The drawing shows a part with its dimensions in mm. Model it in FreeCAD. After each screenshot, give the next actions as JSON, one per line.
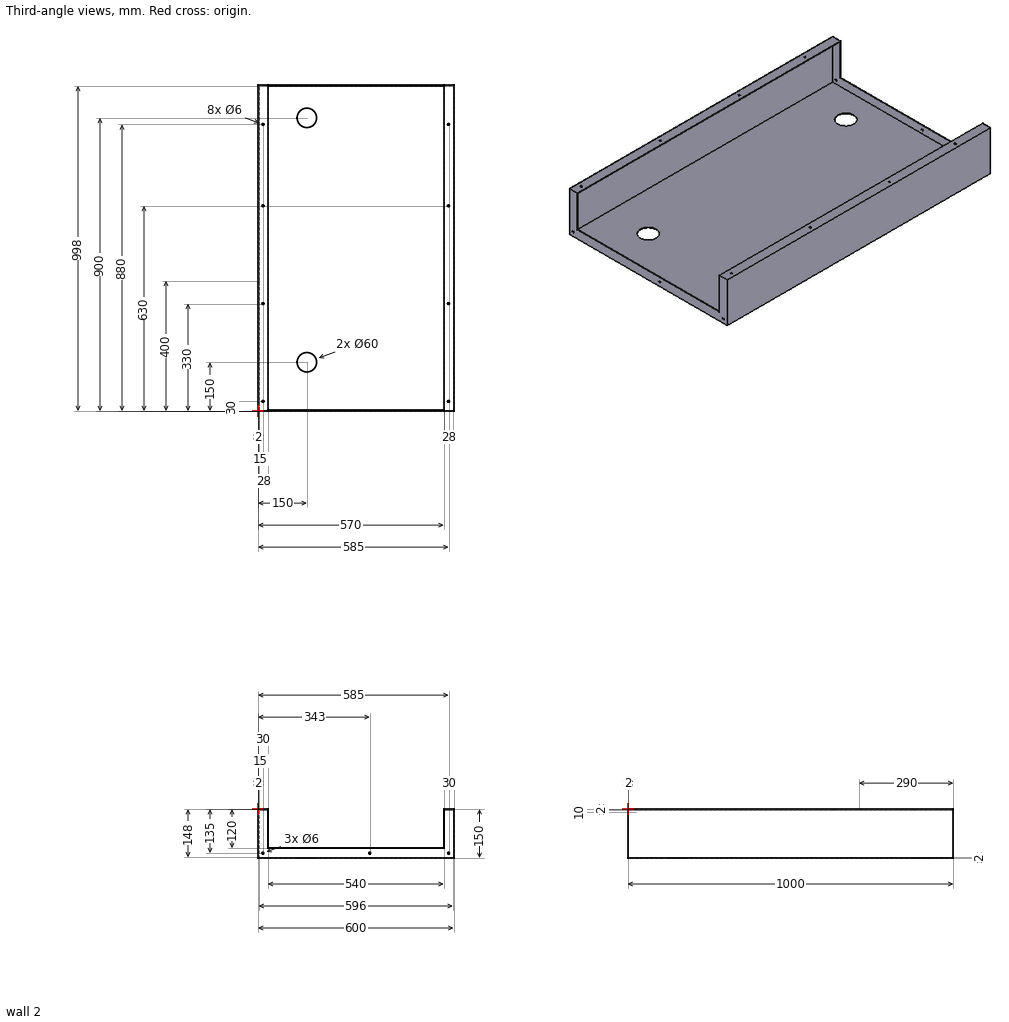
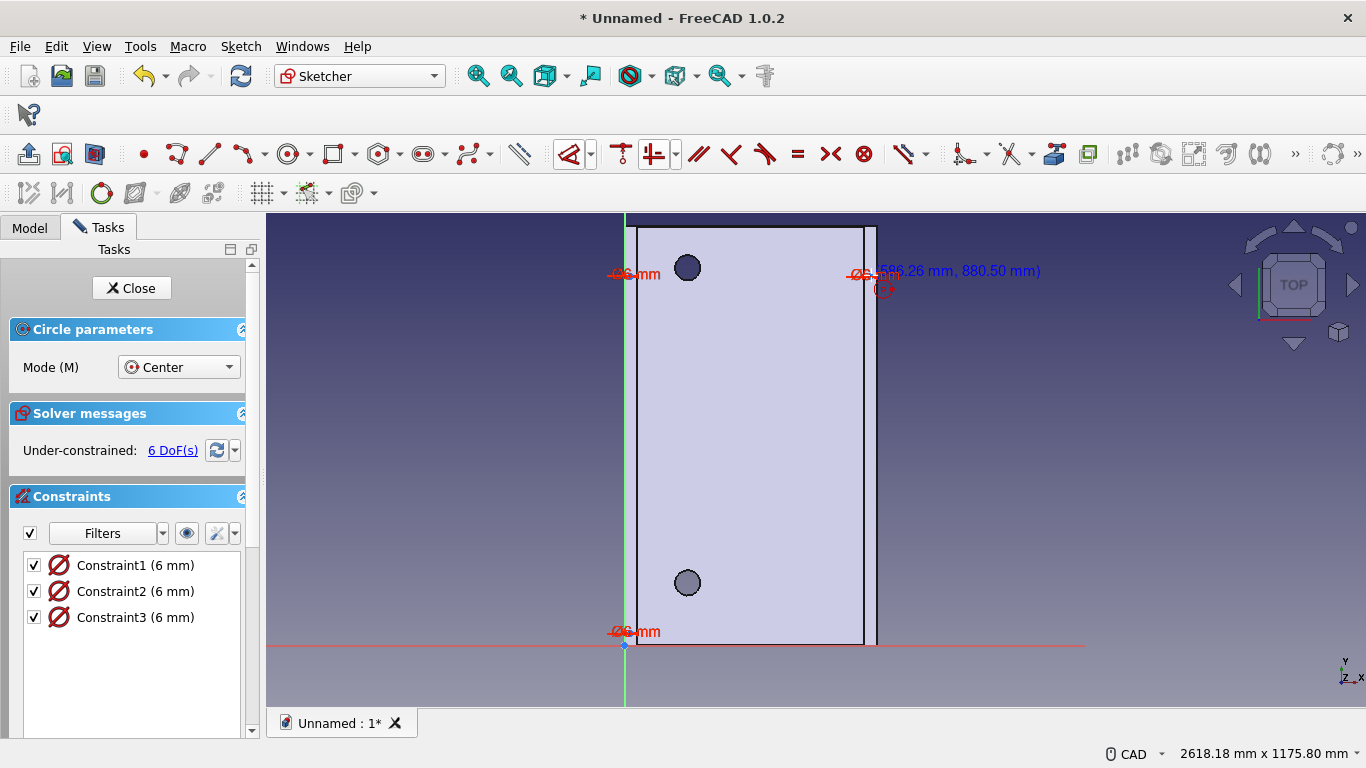
{"action": "scroll", "coordinate": [631, 507], "scroll_direction": "up", "scroll_amount": 15}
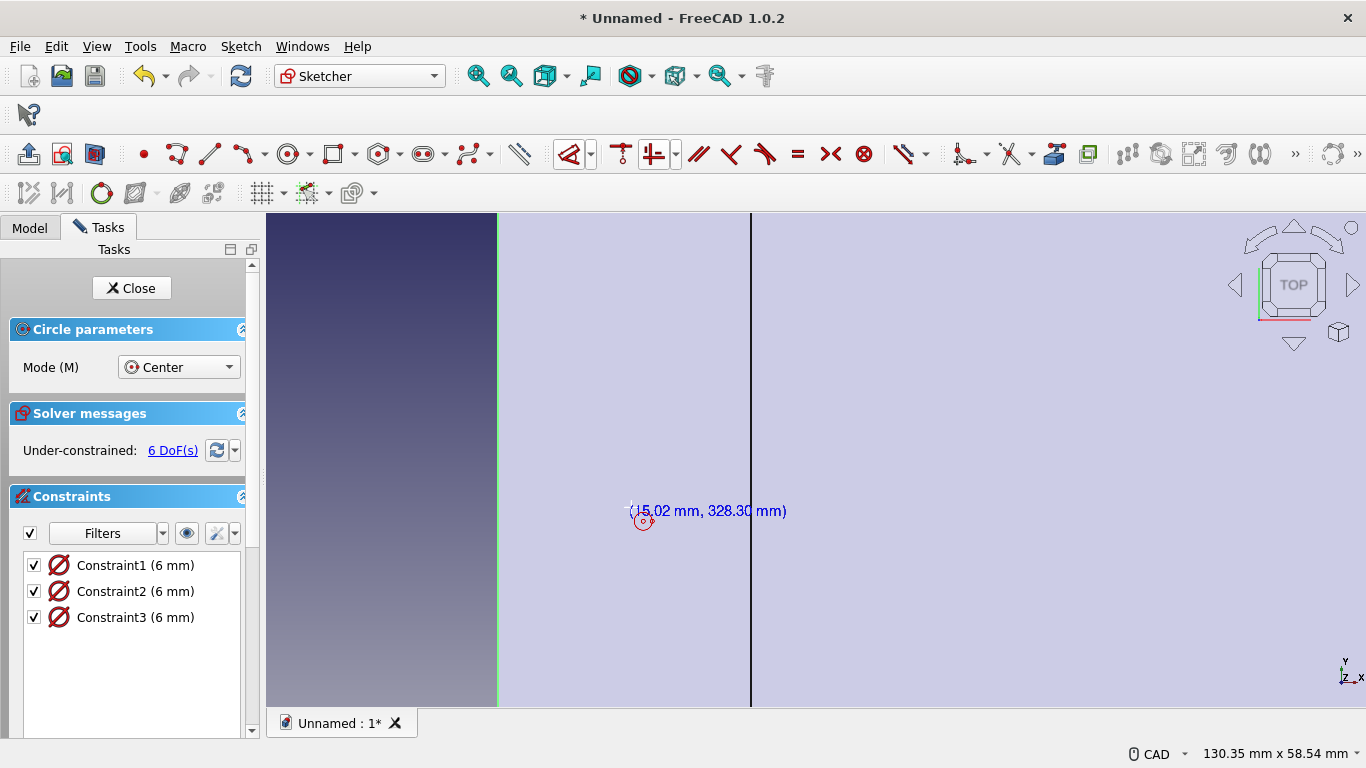
{"action": "scroll", "coordinate": [631, 507], "scroll_direction": "down", "scroll_amount": 15}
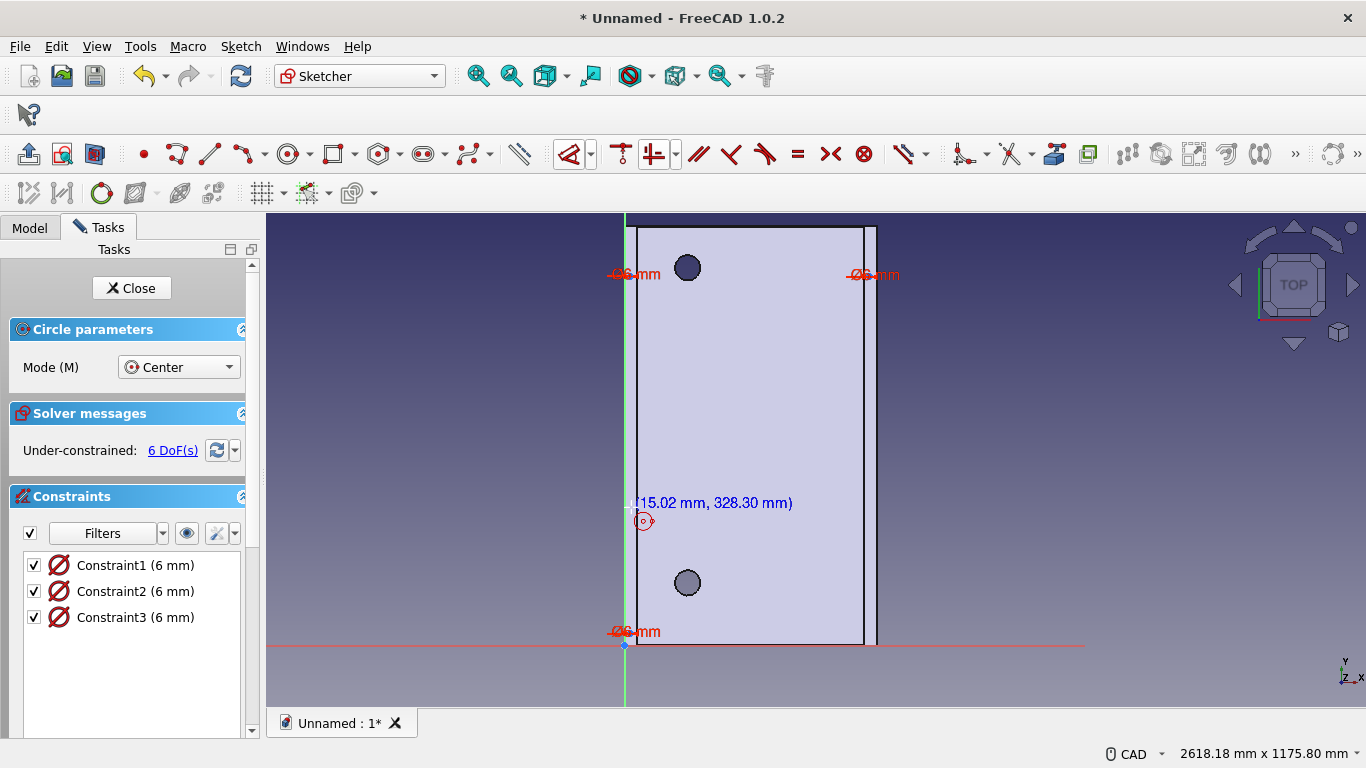
{"action": "scroll", "coordinate": [631, 507], "scroll_direction": "up", "scroll_amount": 5}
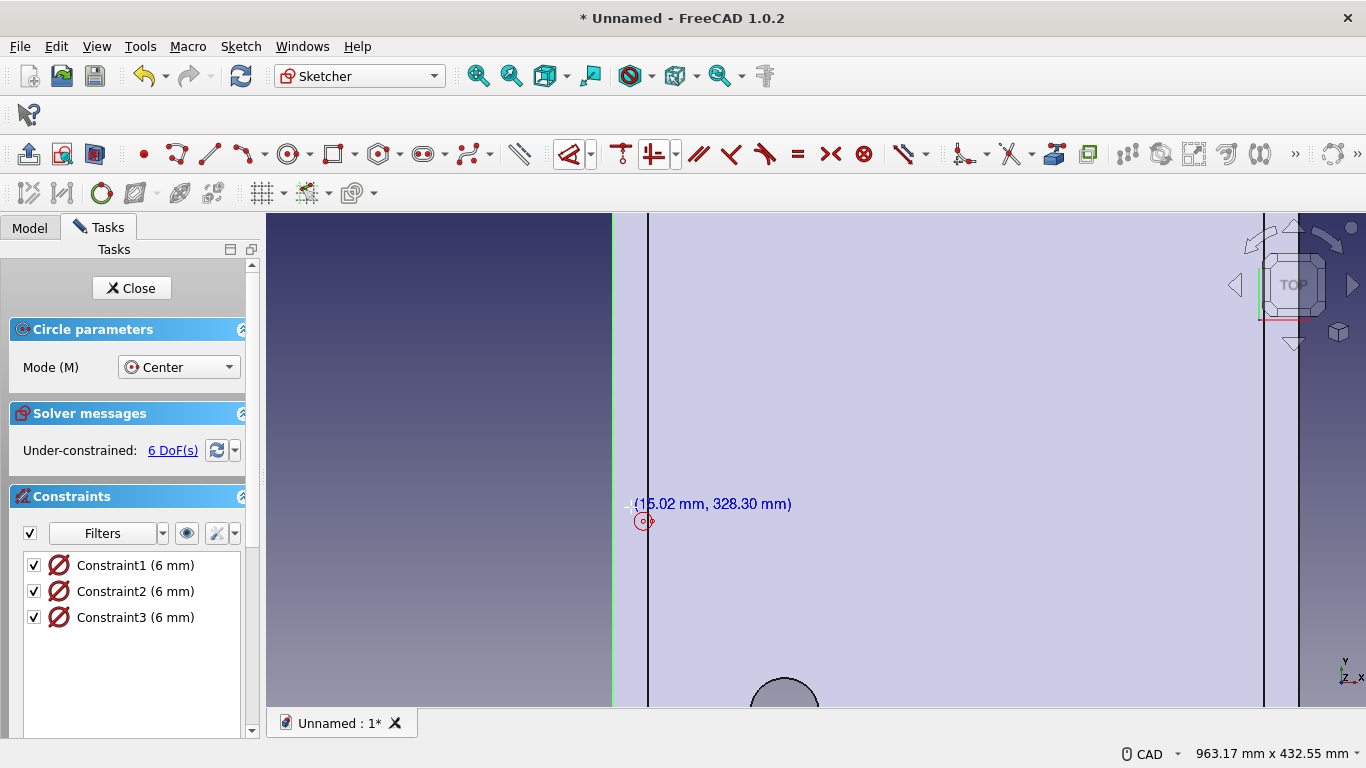
{"action": "left_click", "coordinate": [630, 507]}
{"action": "mouse_move", "coordinate": [633, 504]}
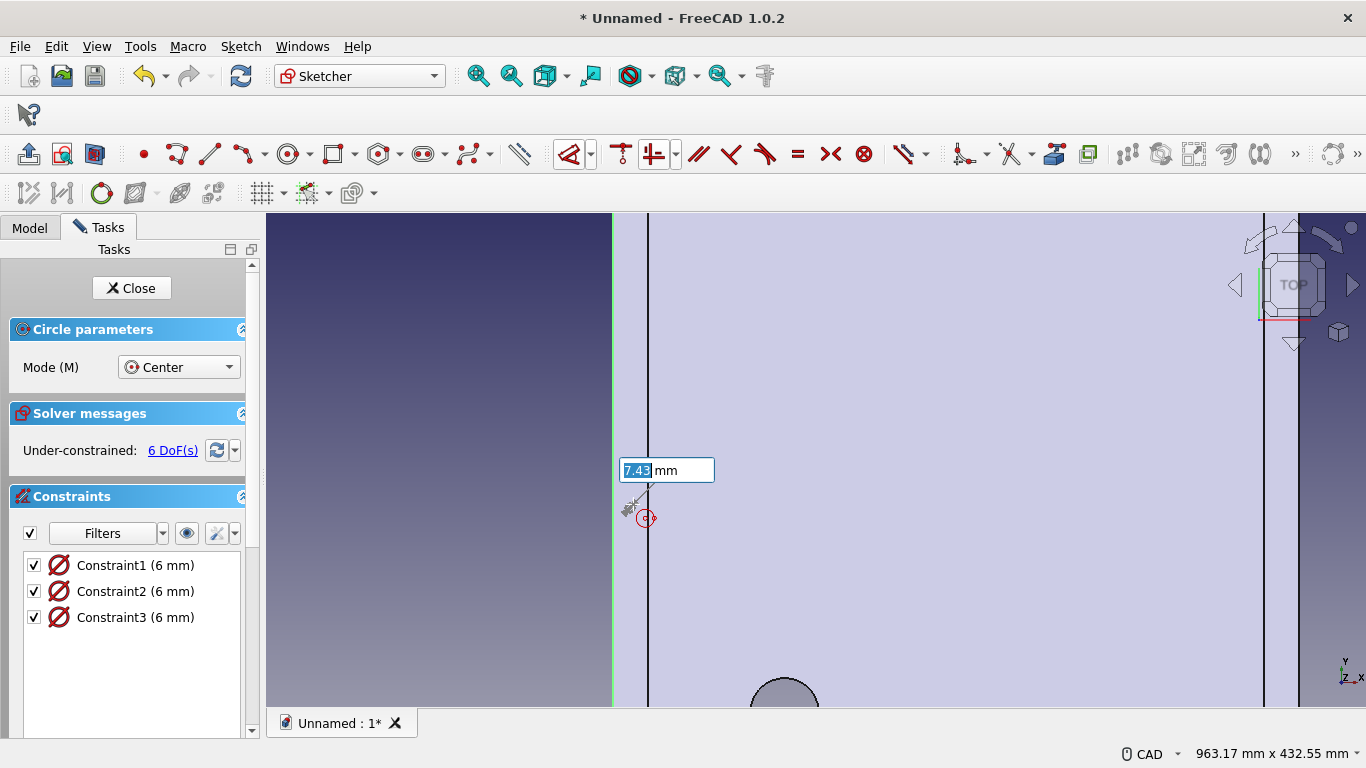
{"action": "type", "text": "6"}
{"action": "key", "text": "Return"}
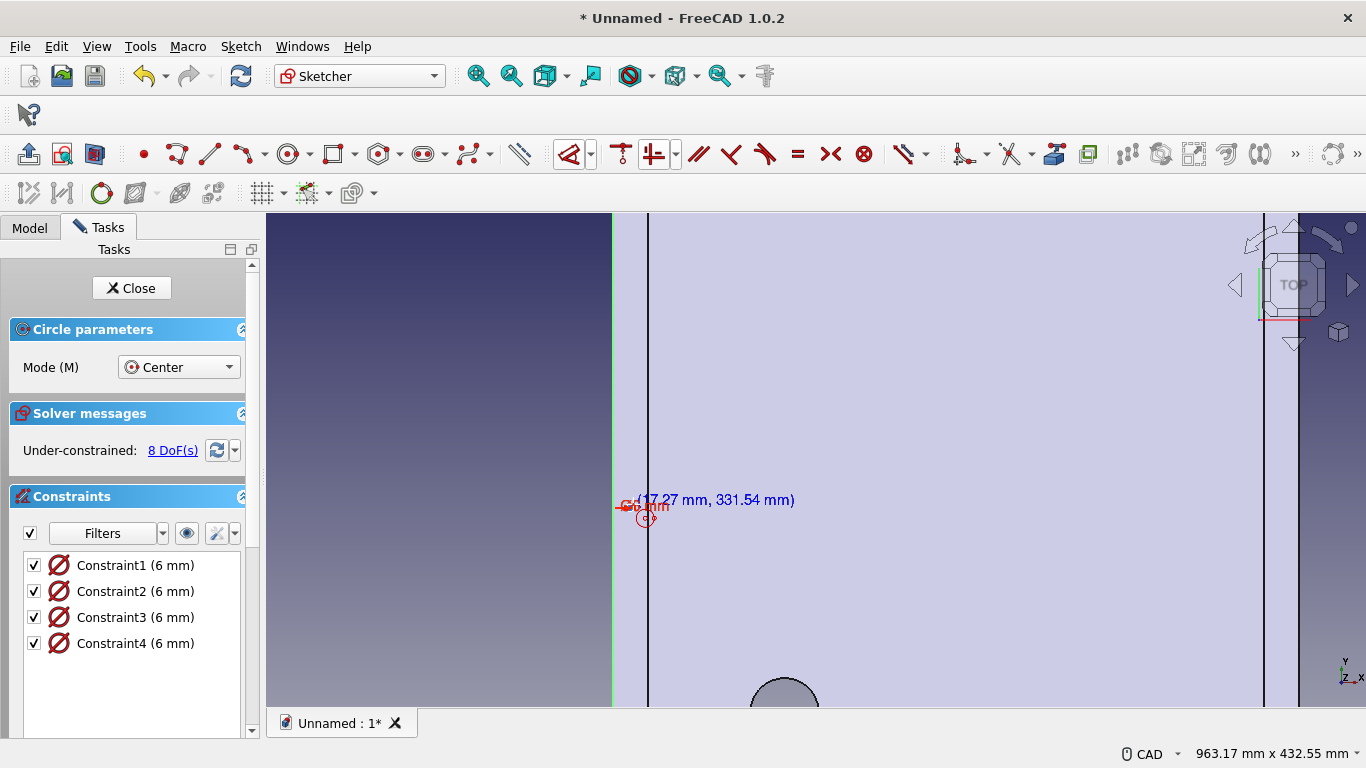
{"action": "scroll", "coordinate": [661, 495], "scroll_direction": "down", "scroll_amount": 6}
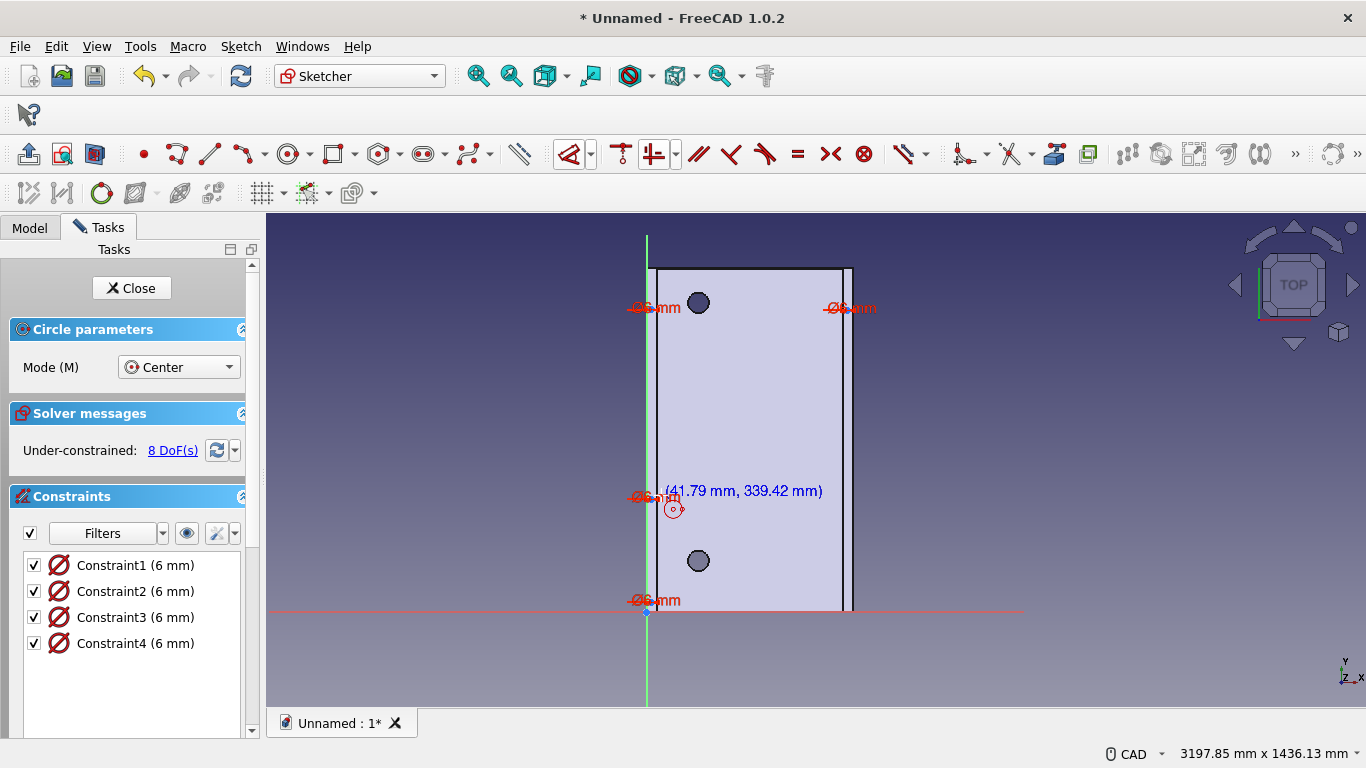
{"action": "scroll", "coordinate": [848, 396], "scroll_direction": "up", "scroll_amount": 16}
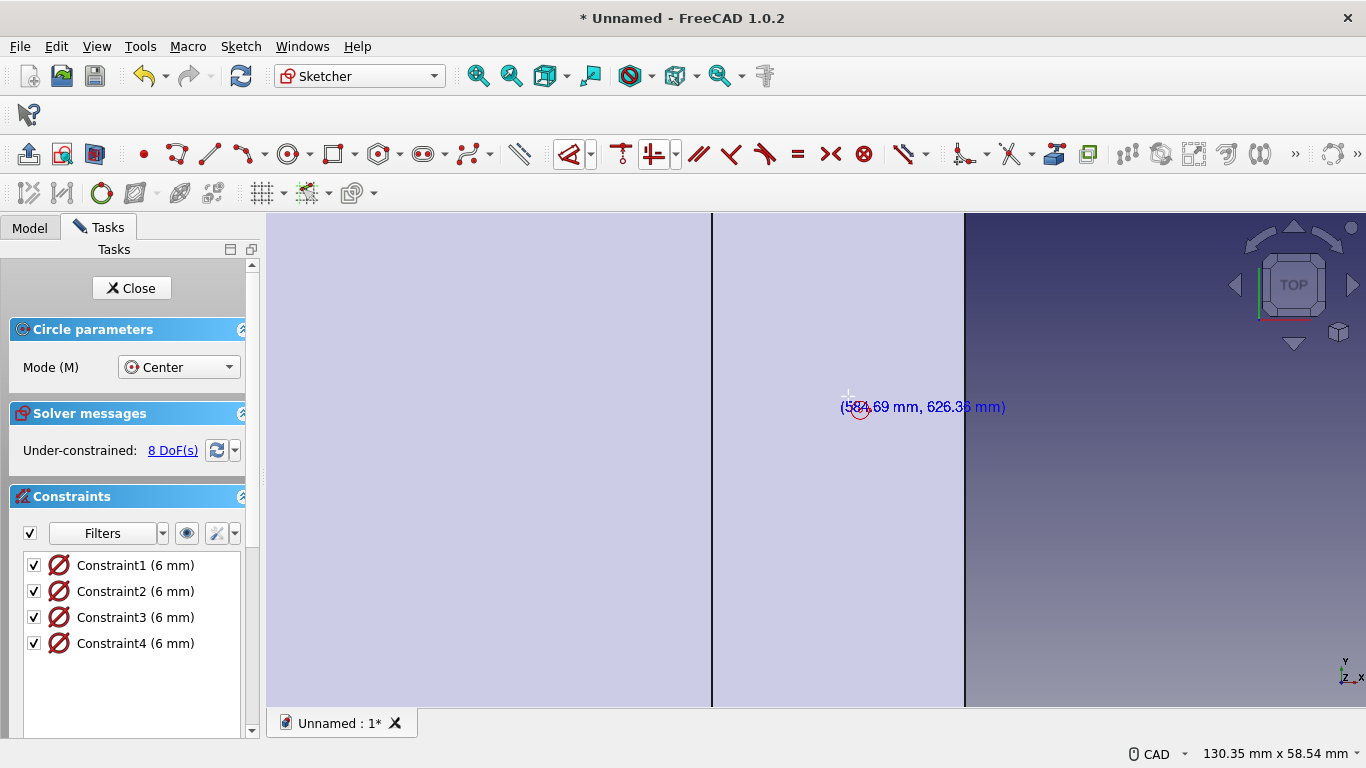
{"action": "scroll", "coordinate": [871, 381], "scroll_direction": "down", "scroll_amount": 15}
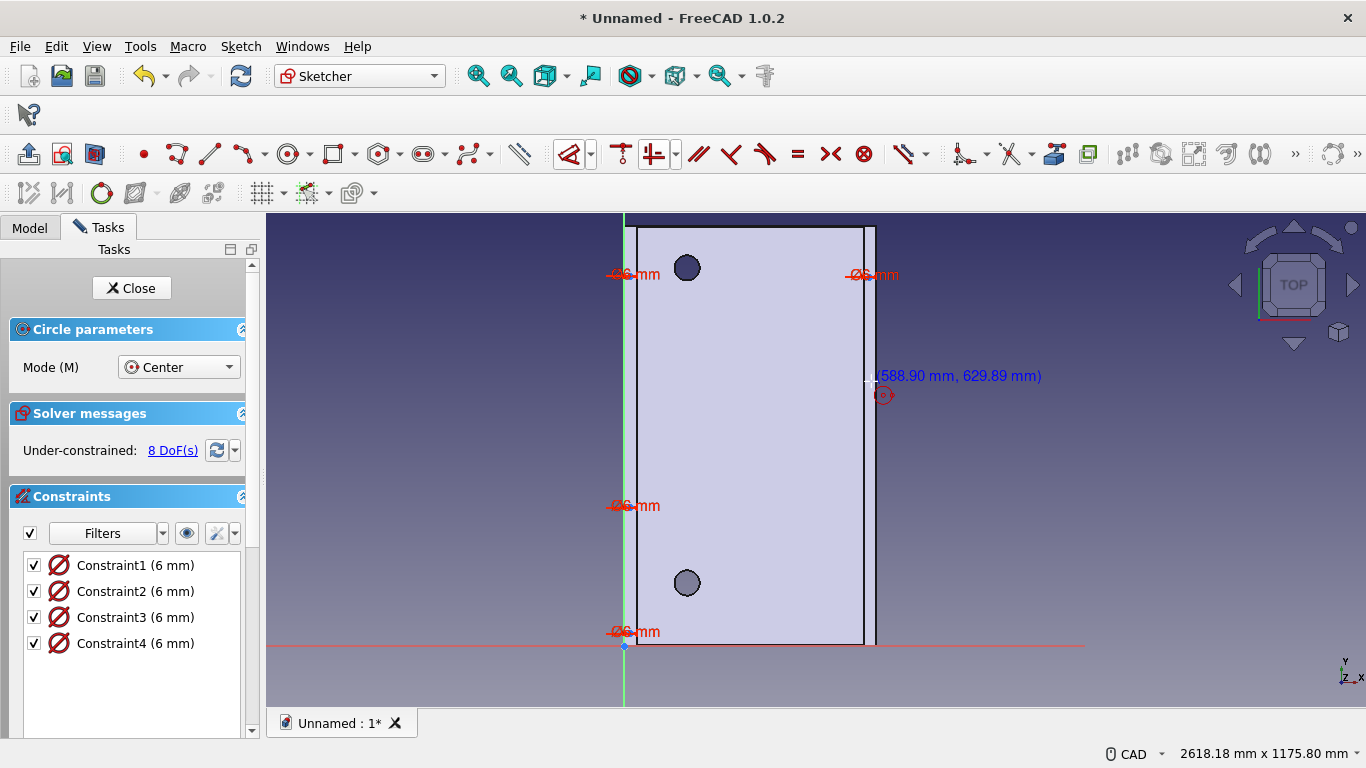
{"action": "left_click", "coordinate": [870, 381]}
{"action": "mouse_move", "coordinate": [871, 380]}